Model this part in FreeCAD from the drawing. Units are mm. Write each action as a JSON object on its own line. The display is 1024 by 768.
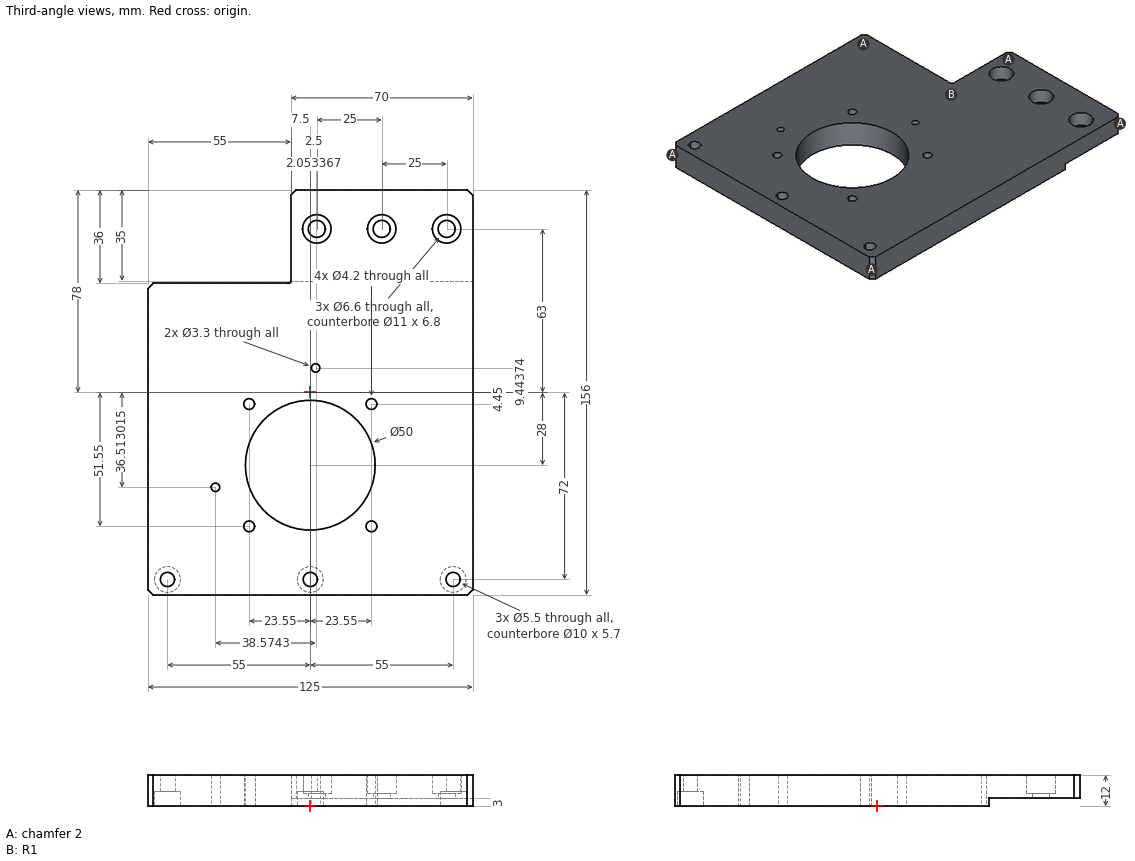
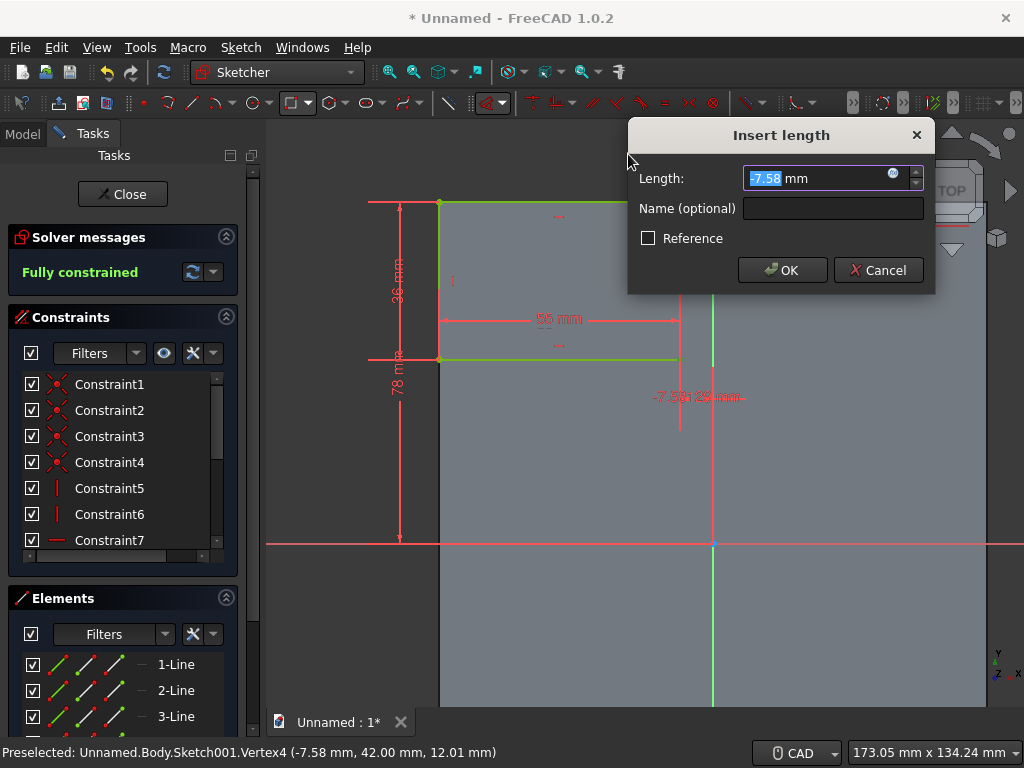
{"action": "type", "text": "-7.5"}
{"action": "key", "text": "Return"}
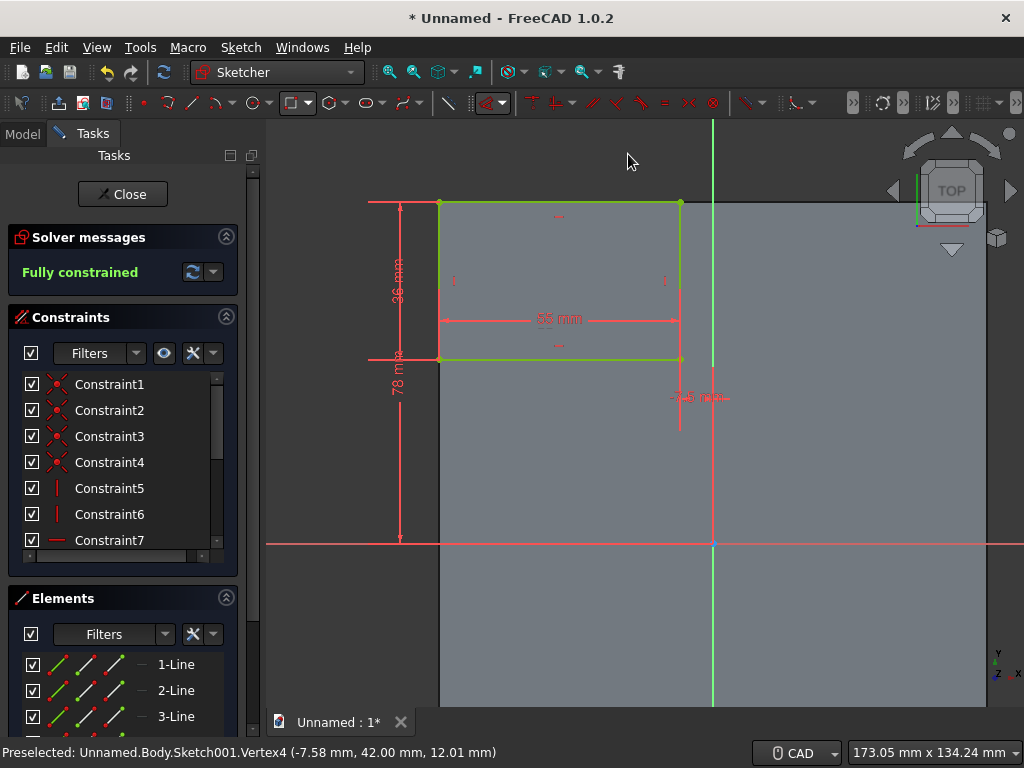
{"action": "left_click", "coordinate": [123, 194]}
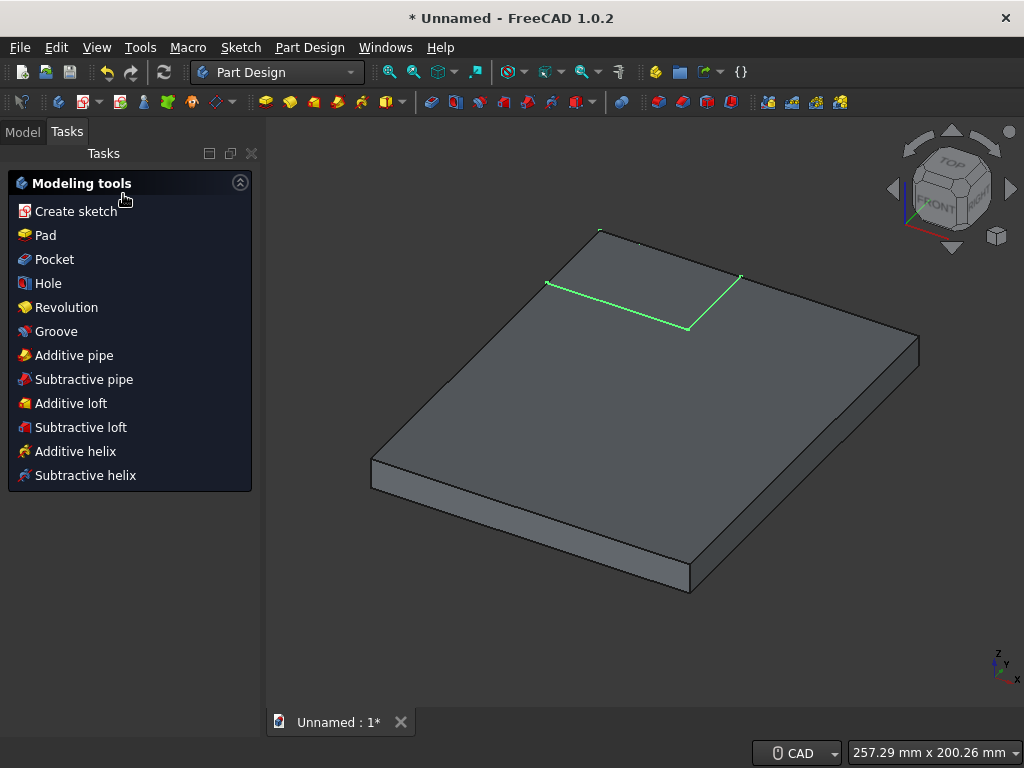
{"action": "left_click", "coordinate": [432, 102]}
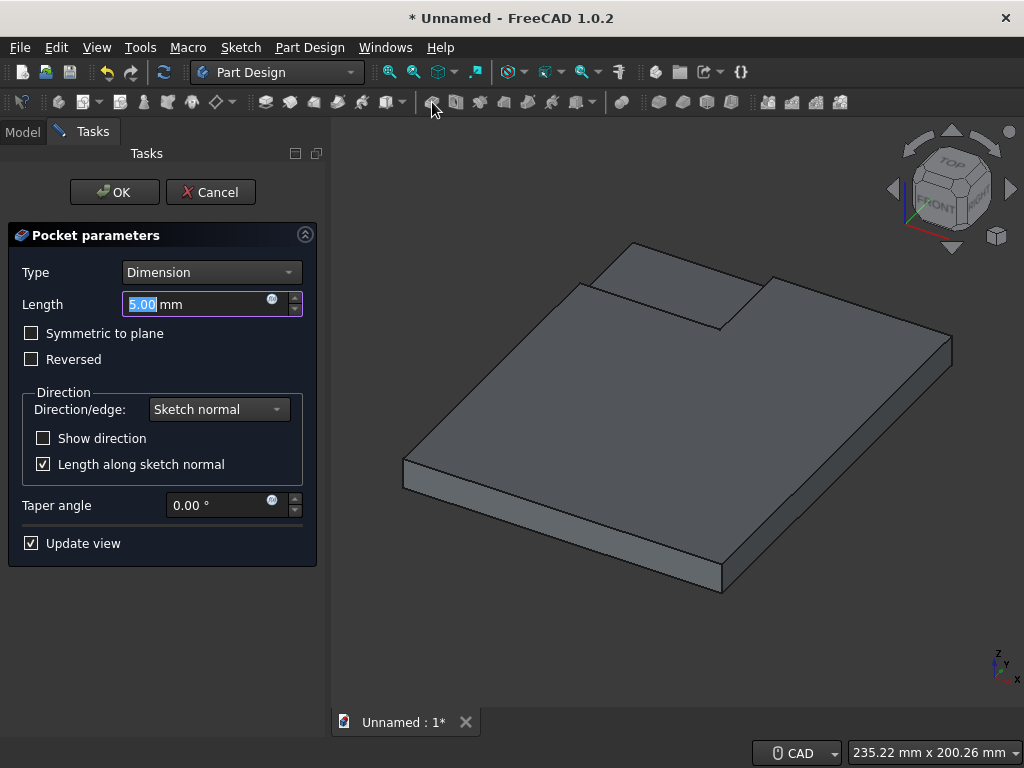
{"action": "left_click", "coordinate": [212, 272]}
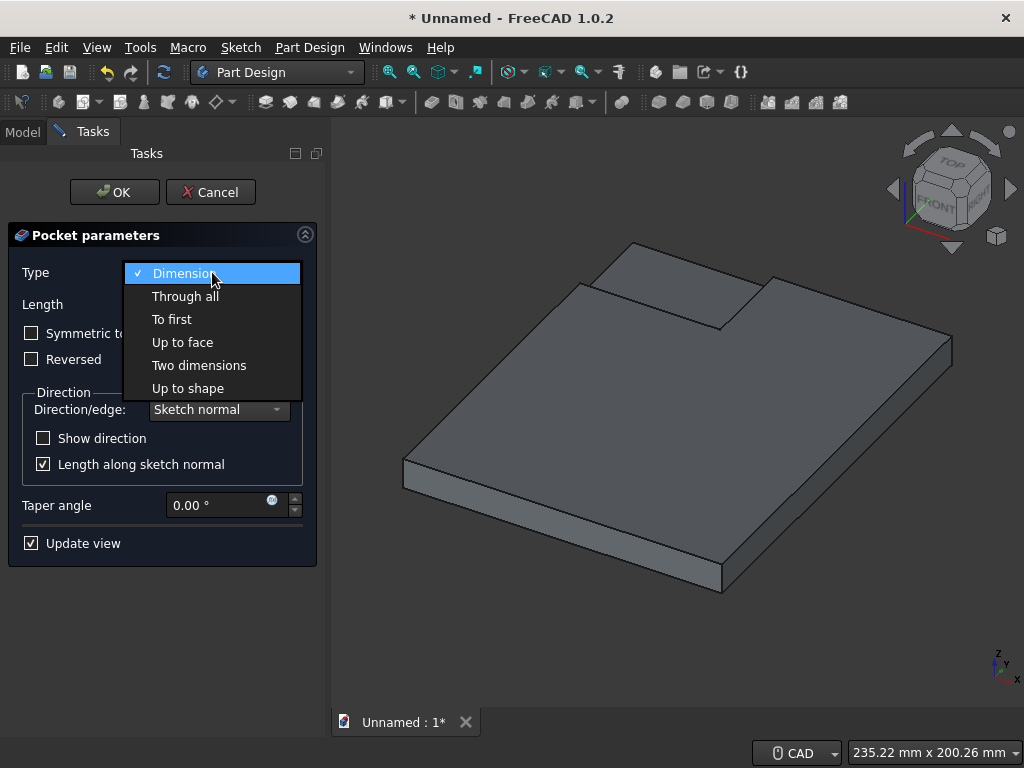
{"action": "left_click", "coordinate": [212, 296]}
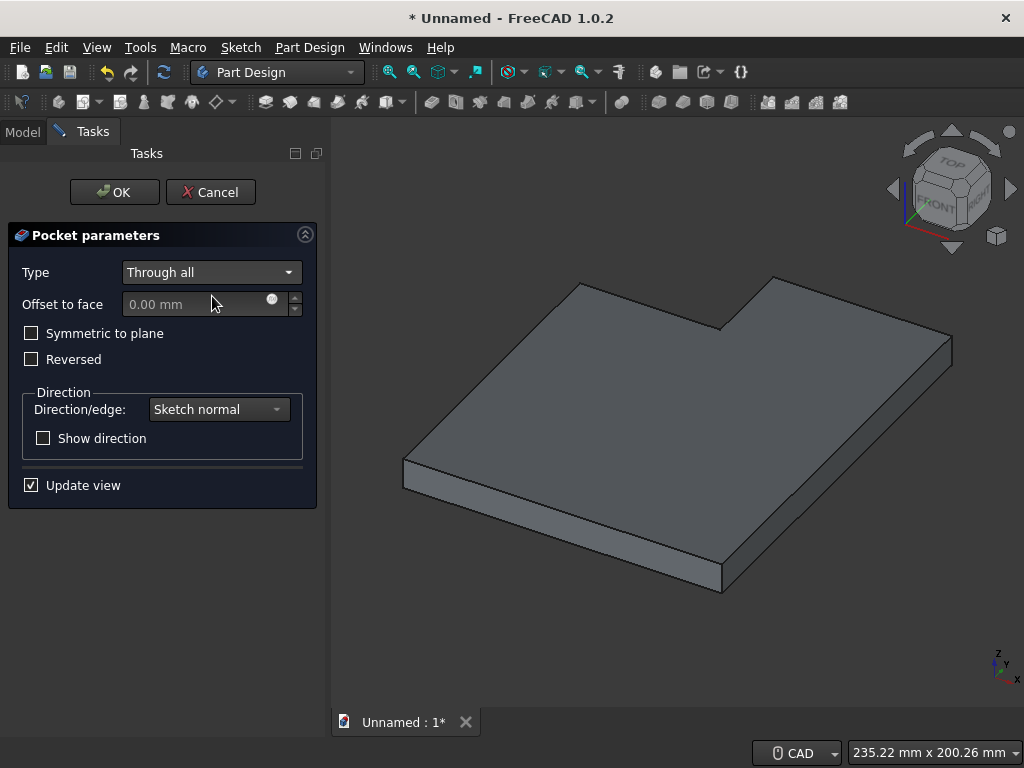
{"action": "left_click", "coordinate": [115, 192]}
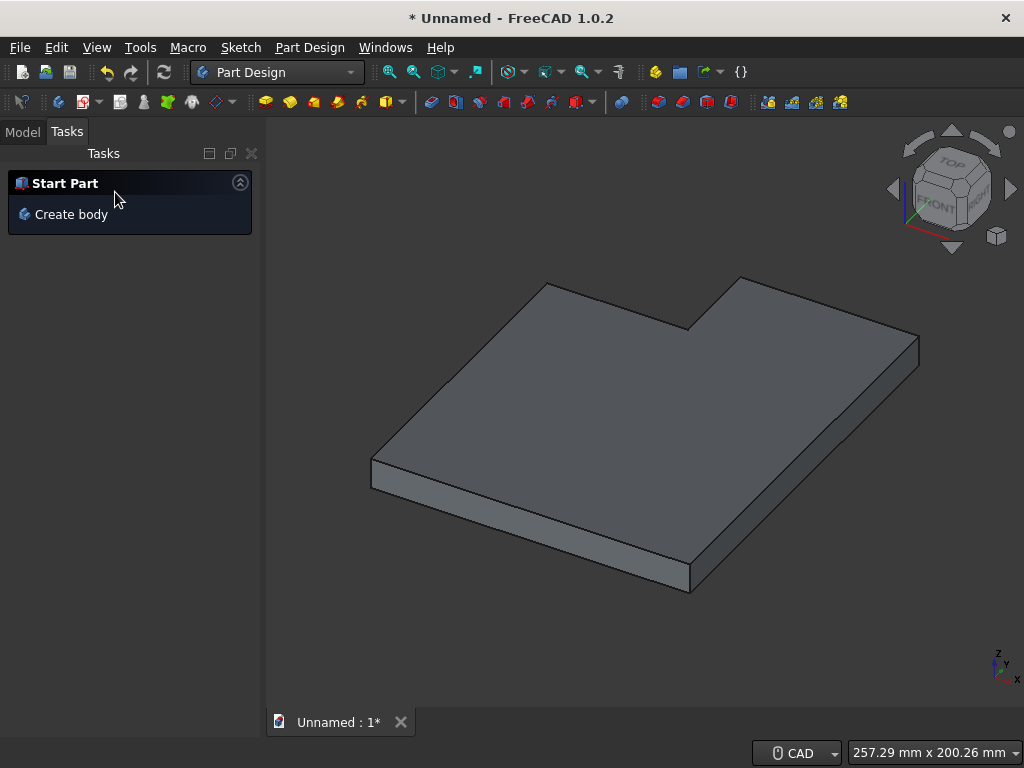
{"action": "left_click", "coordinate": [84, 102]}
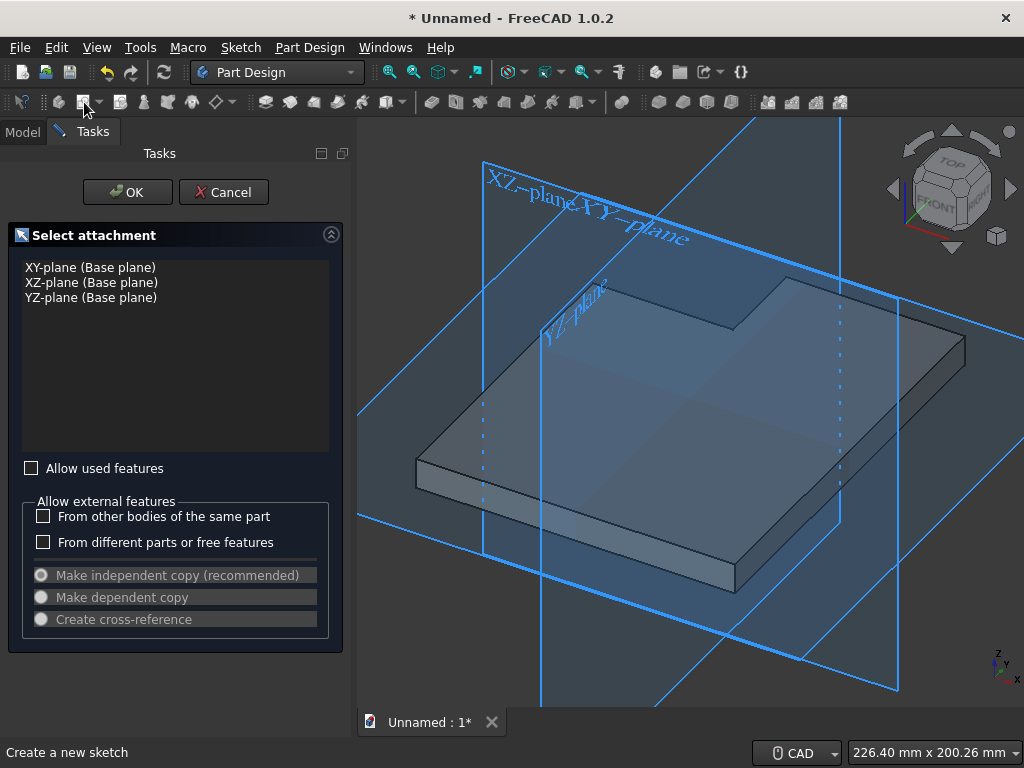
{"action": "left_click", "coordinate": [82, 268]}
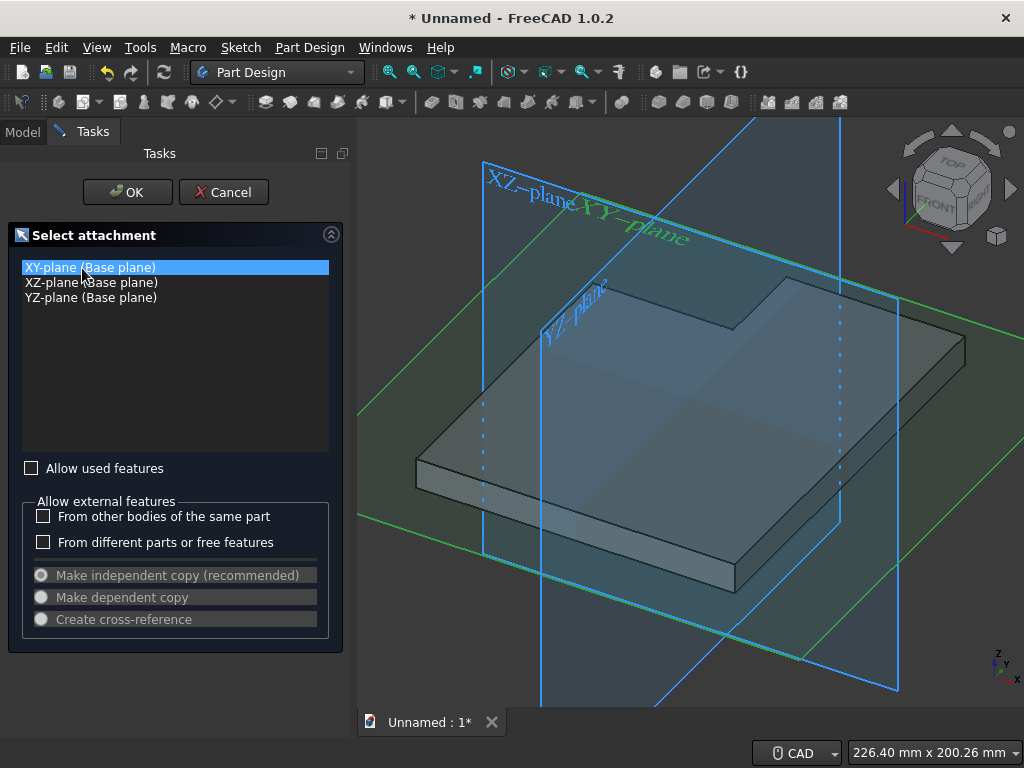
{"action": "left_click", "coordinate": [128, 192]}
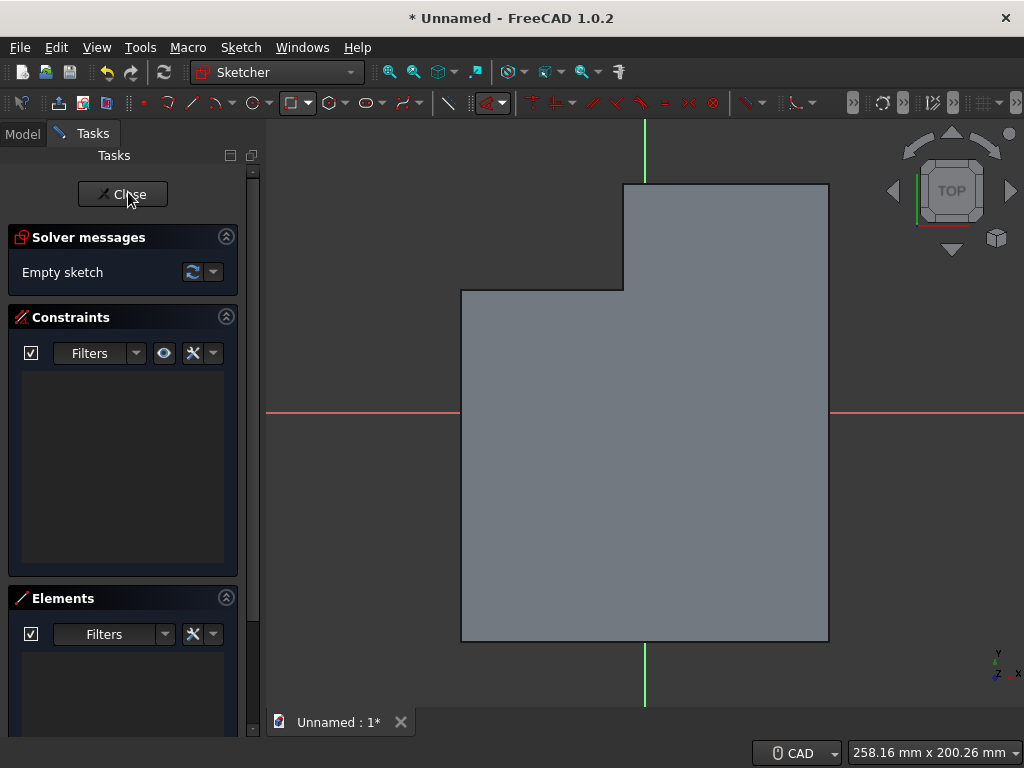
{"action": "left_click", "coordinate": [108, 104]}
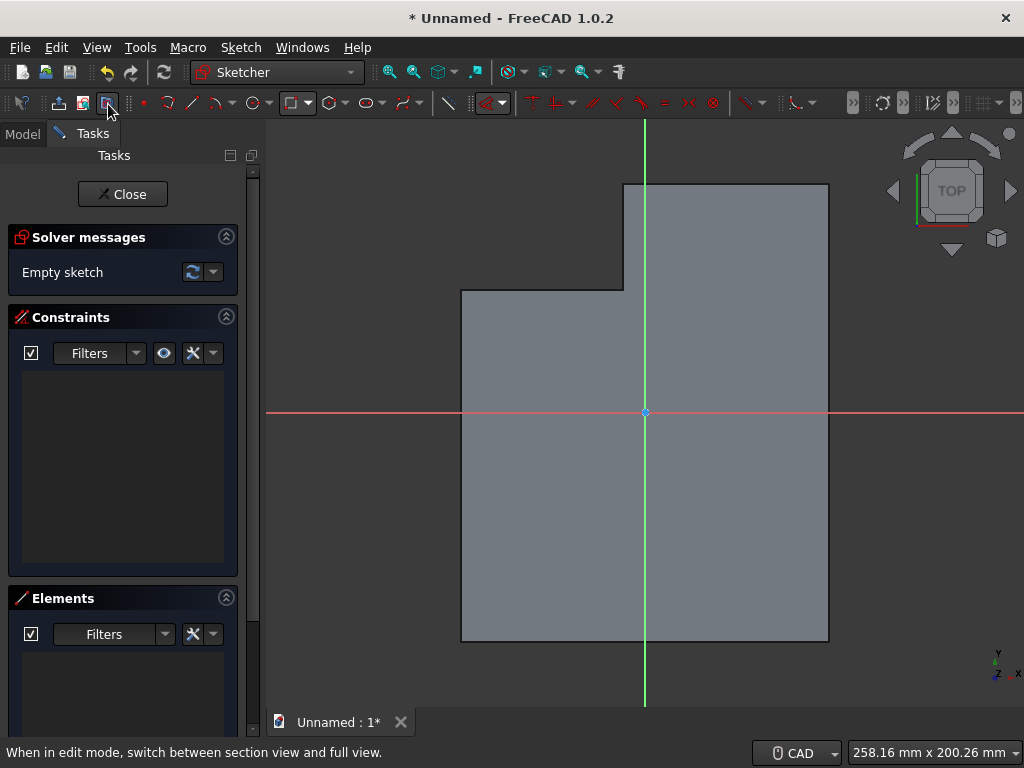
{"action": "scroll", "coordinate": [859, 147], "scroll_direction": "up", "scroll_amount": 2}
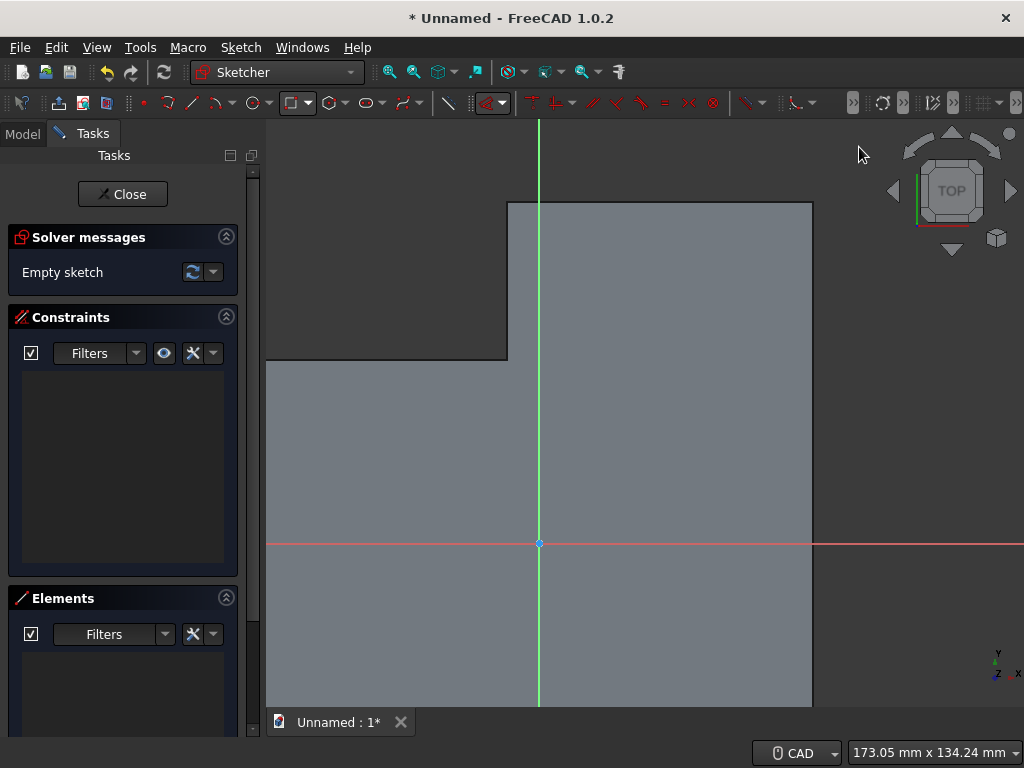
{"action": "left_click", "coordinate": [292, 104]}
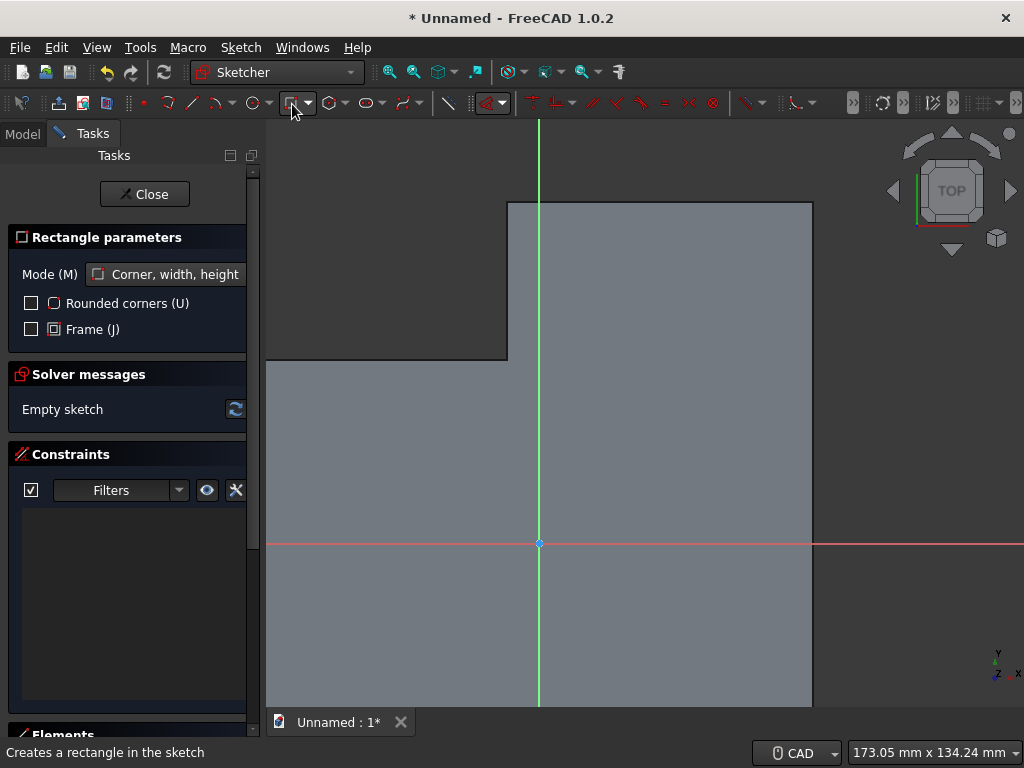
{"action": "left_click", "coordinate": [507, 202]}
{"action": "left_click", "coordinate": [813, 355]}
{"action": "key", "text": "Escape"}